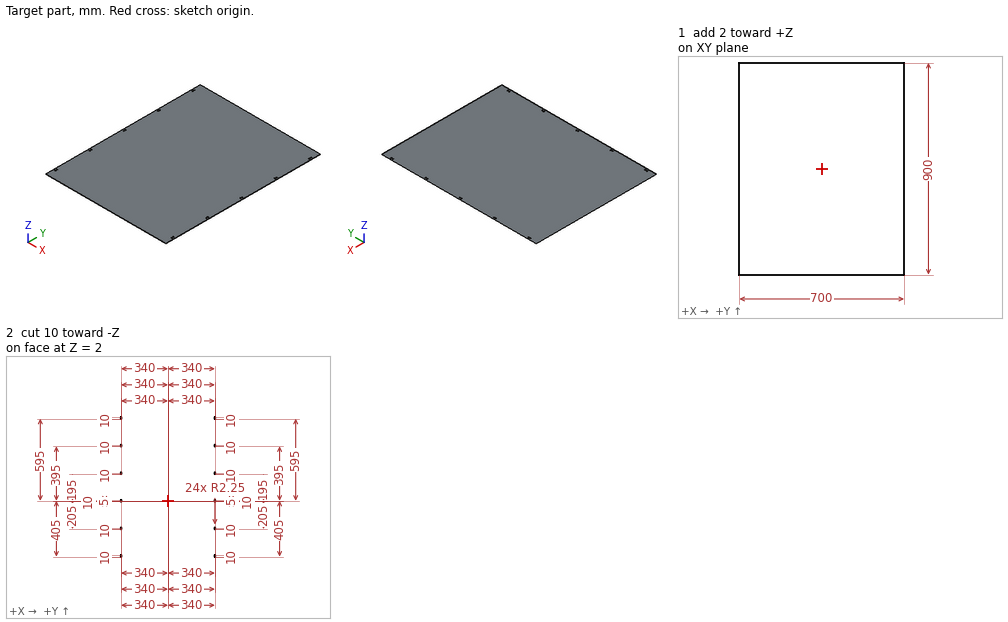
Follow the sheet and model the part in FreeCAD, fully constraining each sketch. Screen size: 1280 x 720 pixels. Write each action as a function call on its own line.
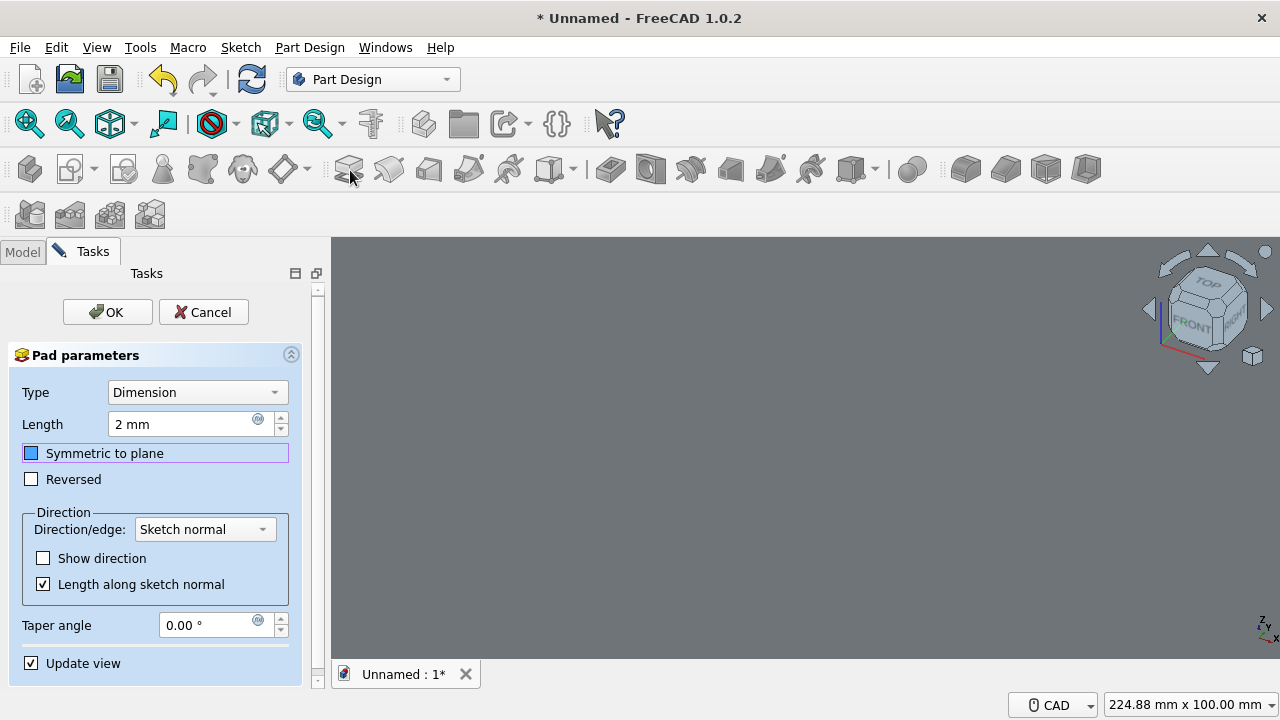
click(108, 312)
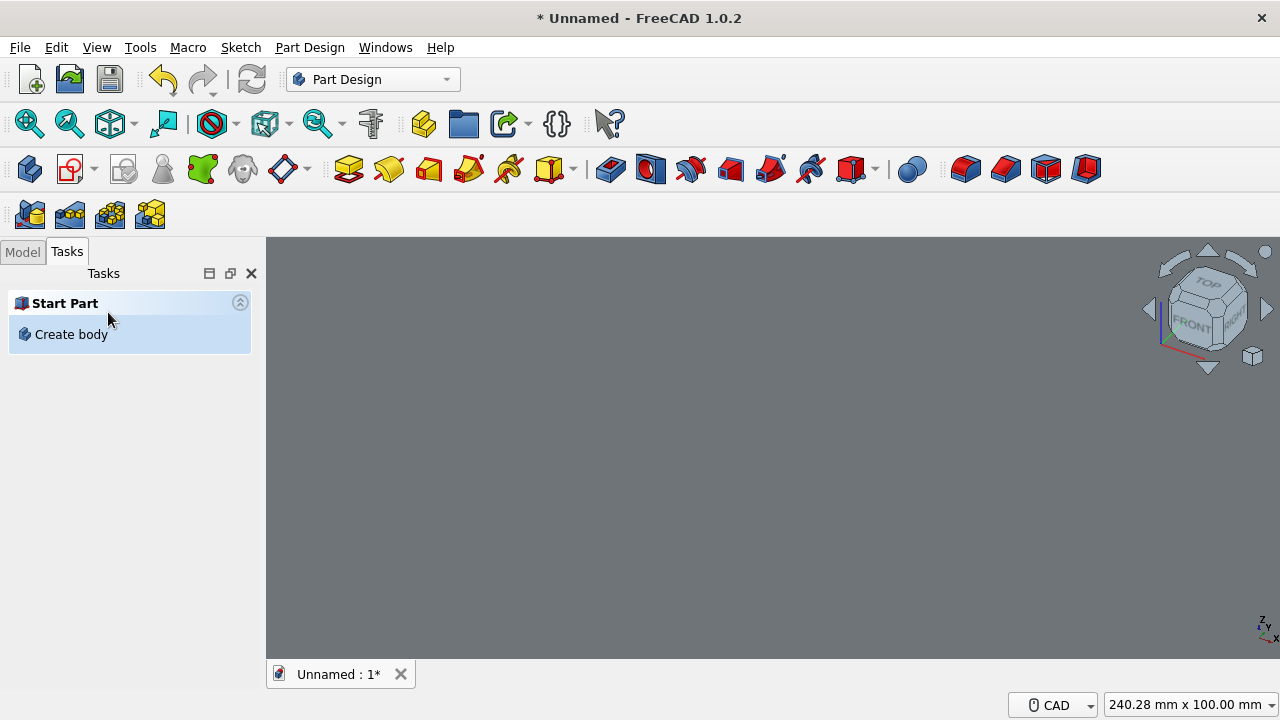
click(30, 124)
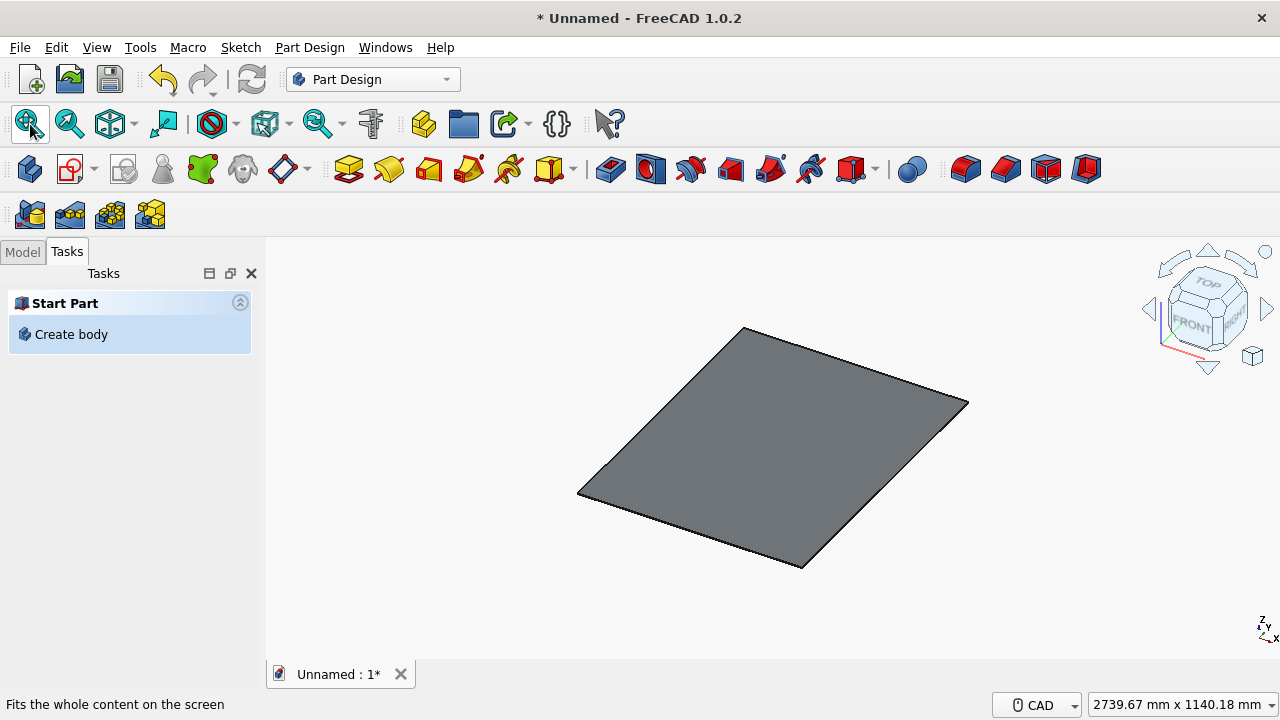
click(773, 447)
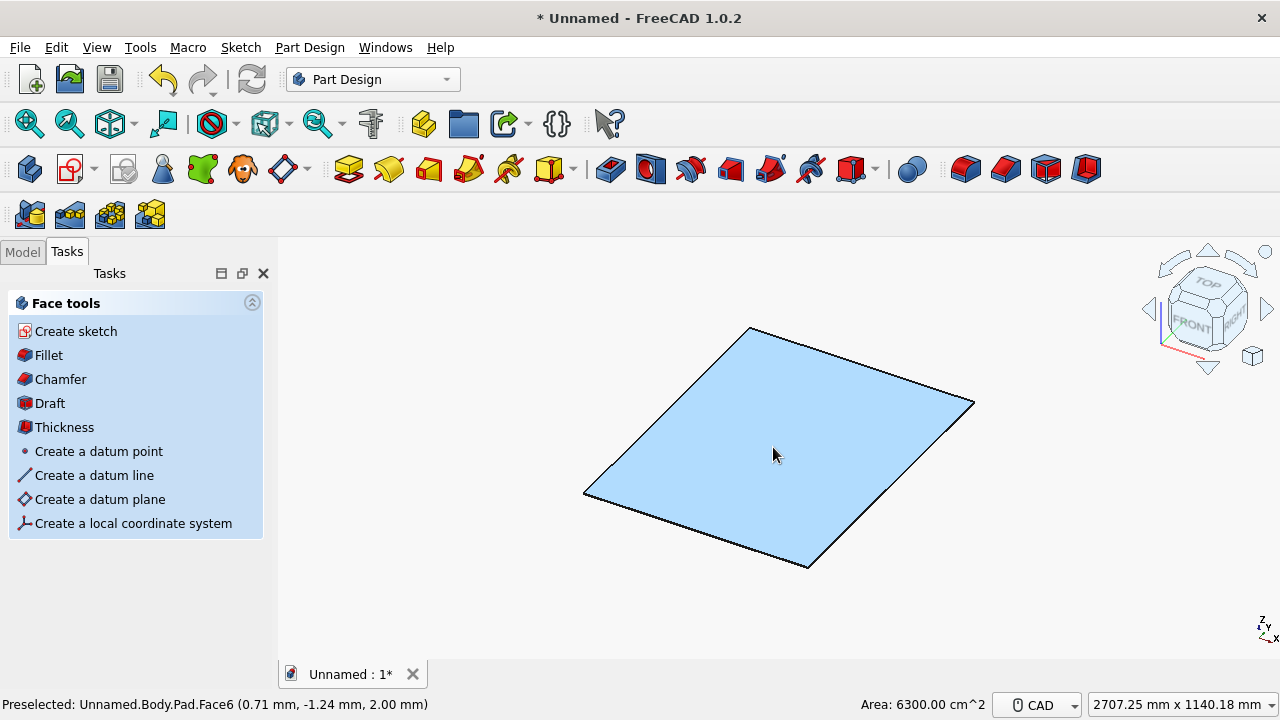
click(70, 170)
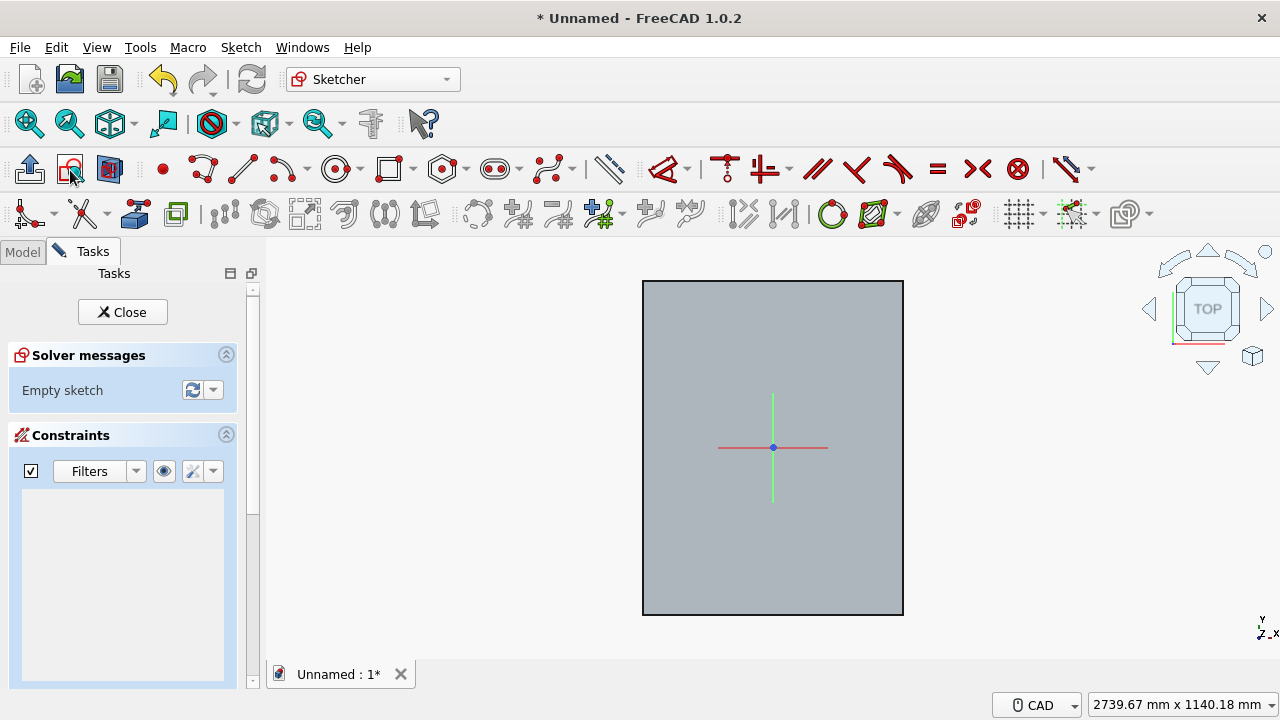
scroll(565, 523, down, 2)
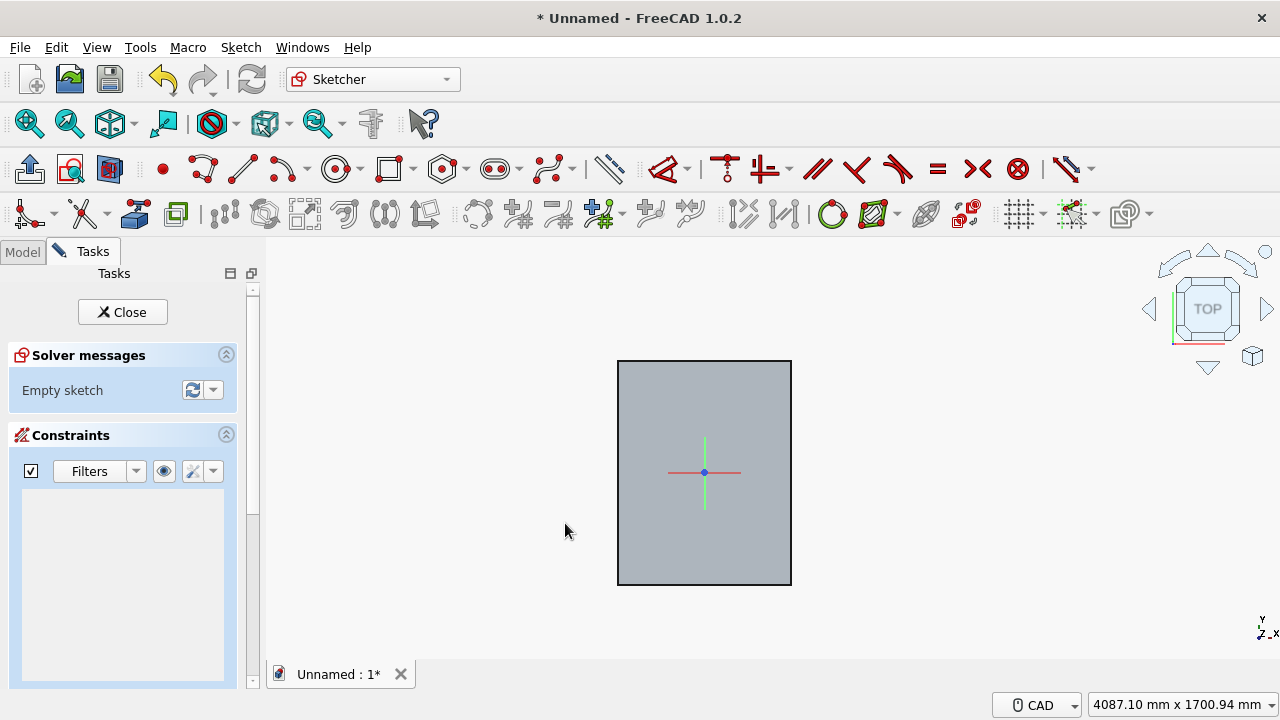
click(496, 170)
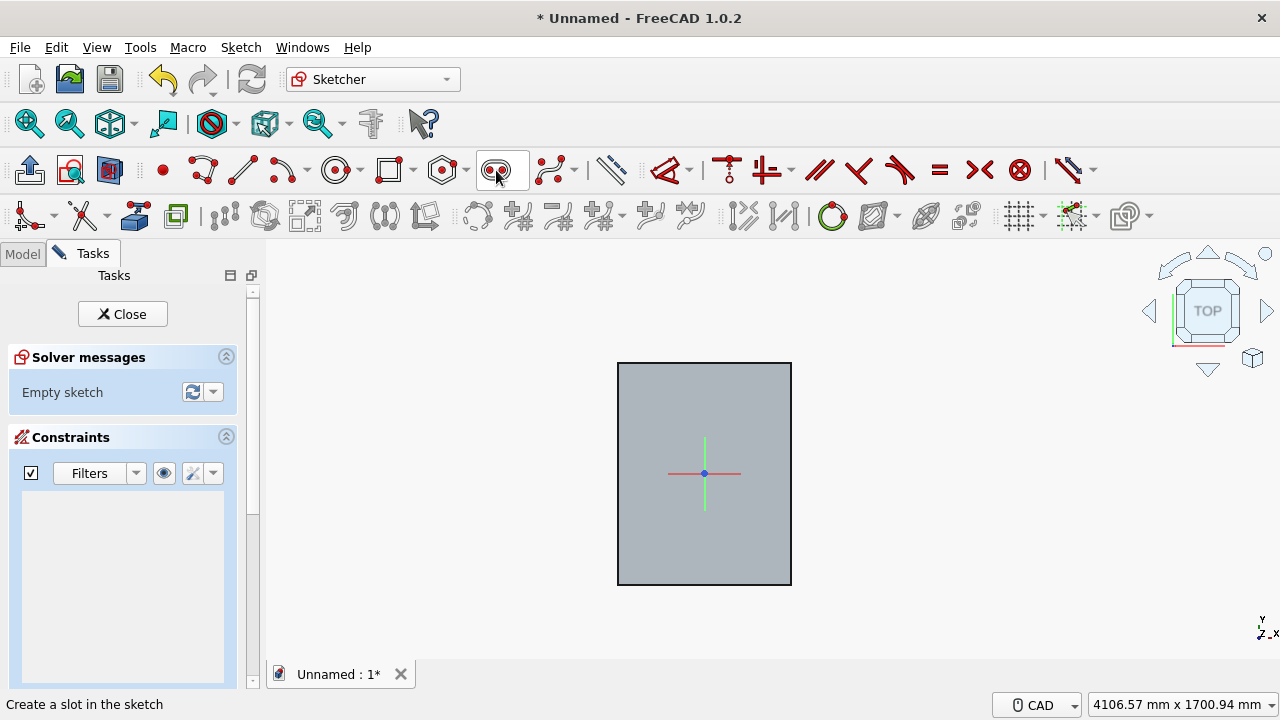
scroll(621, 376, up, 19)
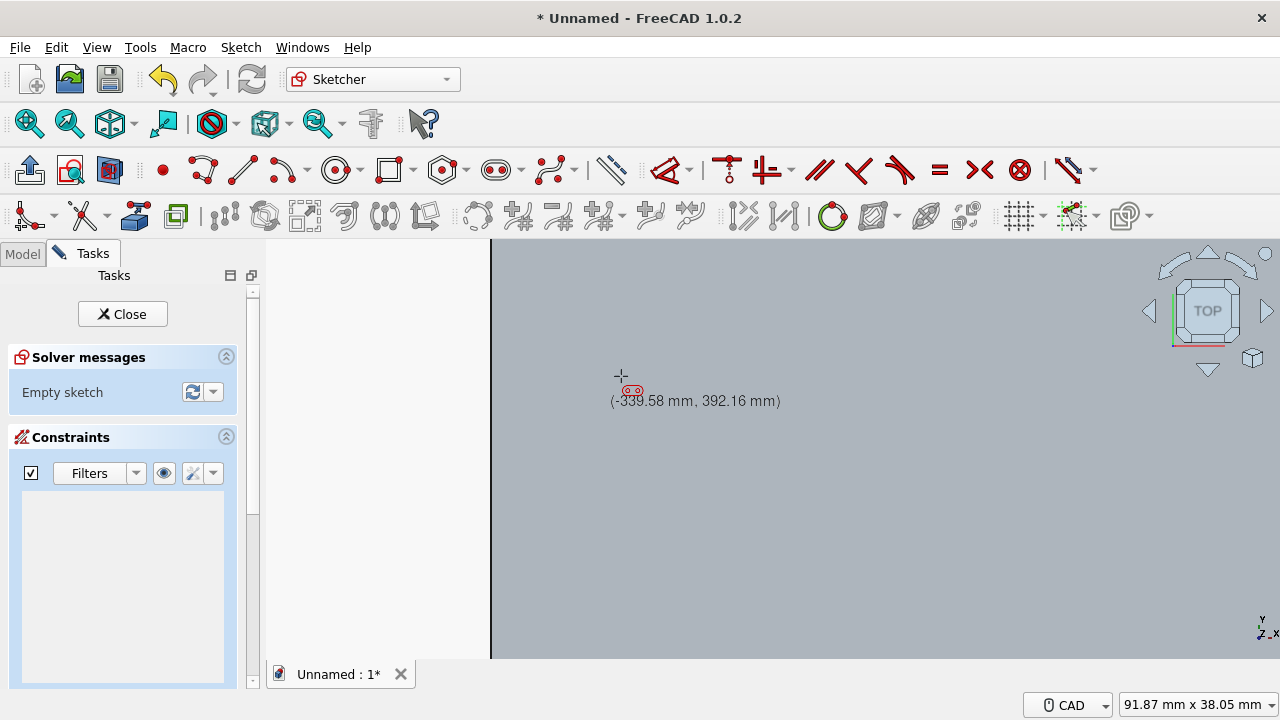
scroll(602, 360, down, 18)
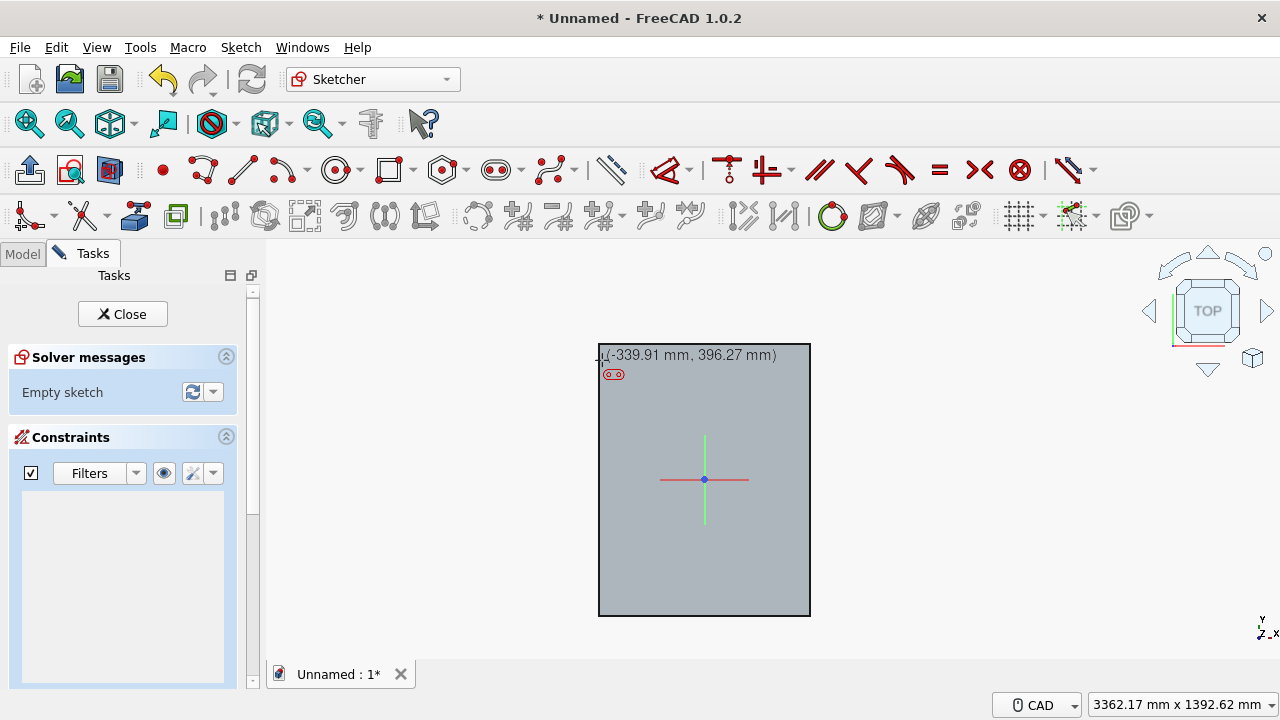
click(602, 361)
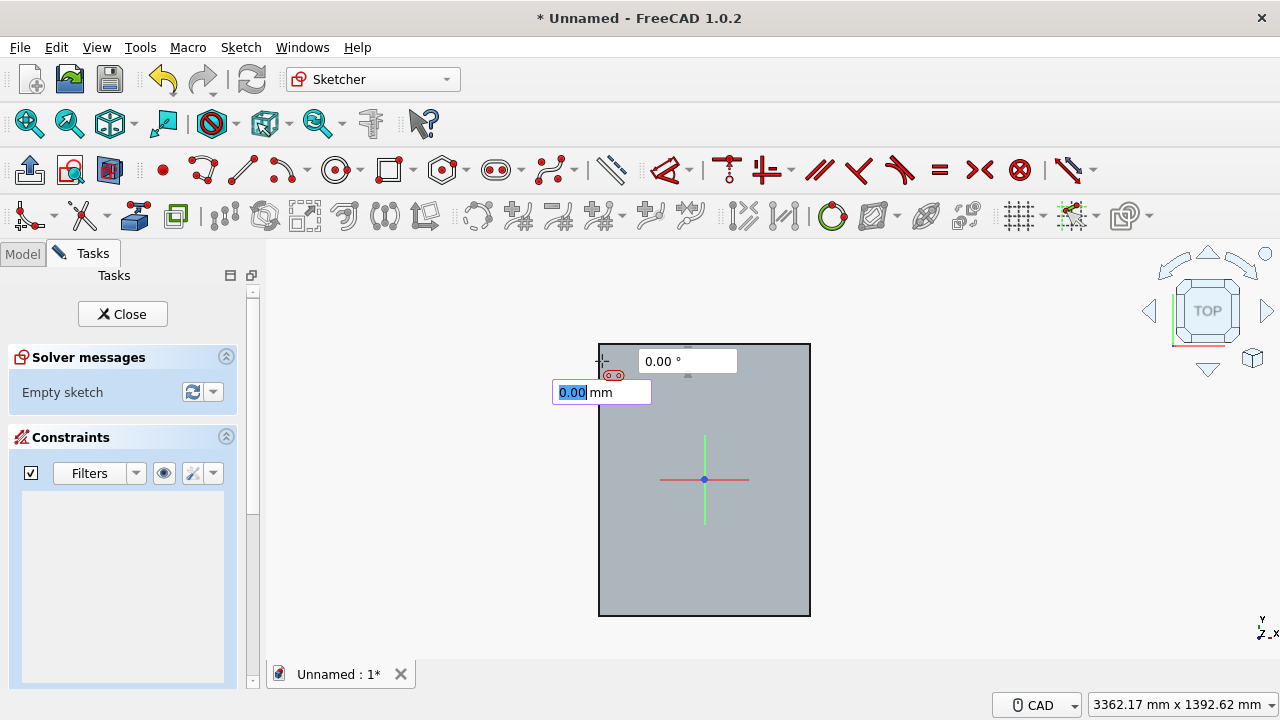
scroll(602, 358, up, 9)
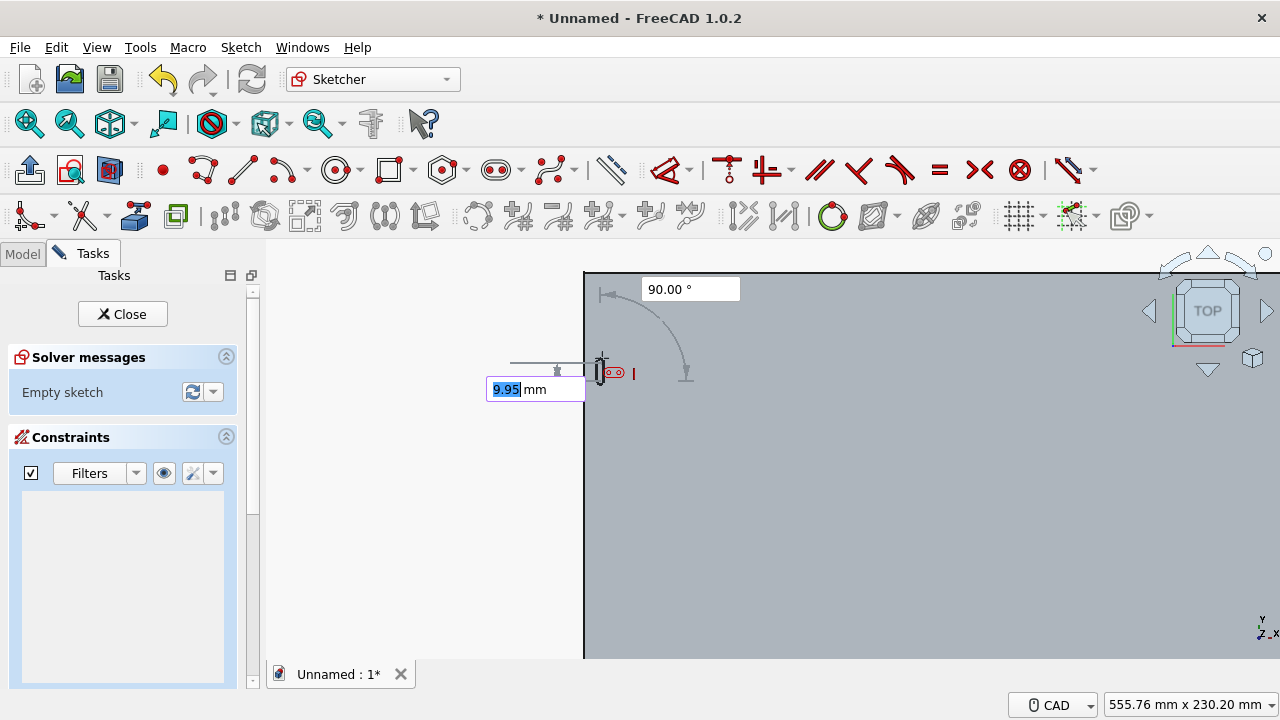
click(600, 355)